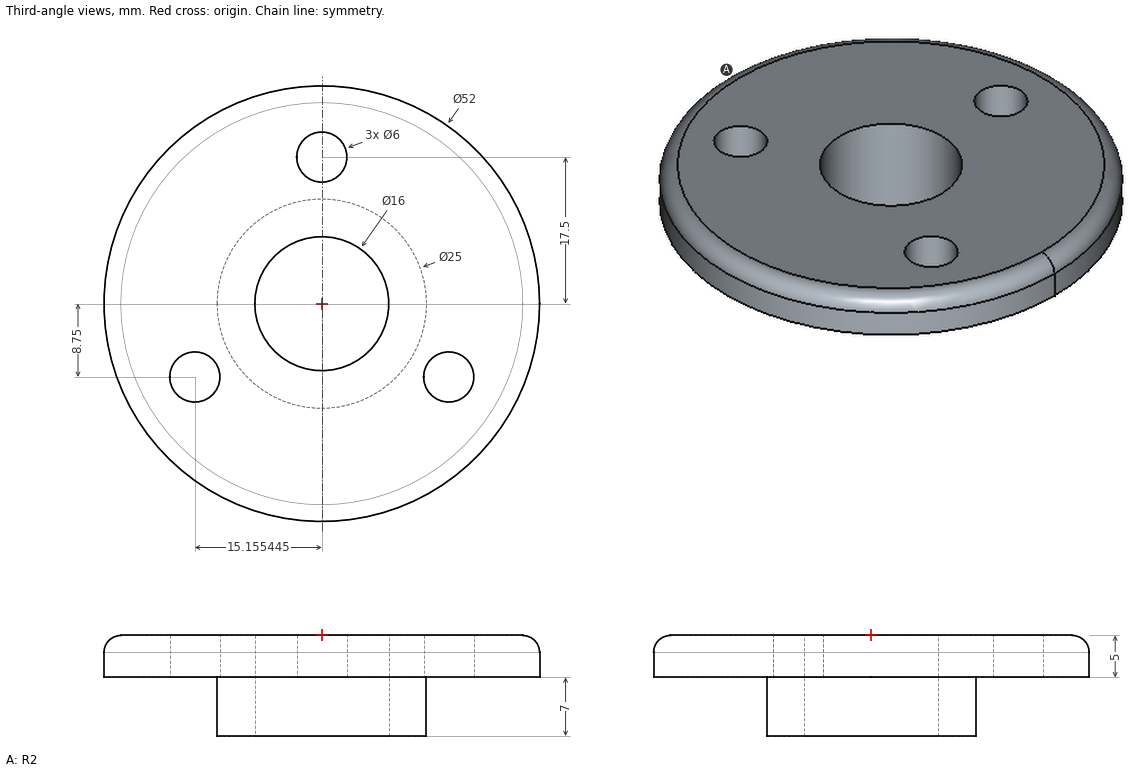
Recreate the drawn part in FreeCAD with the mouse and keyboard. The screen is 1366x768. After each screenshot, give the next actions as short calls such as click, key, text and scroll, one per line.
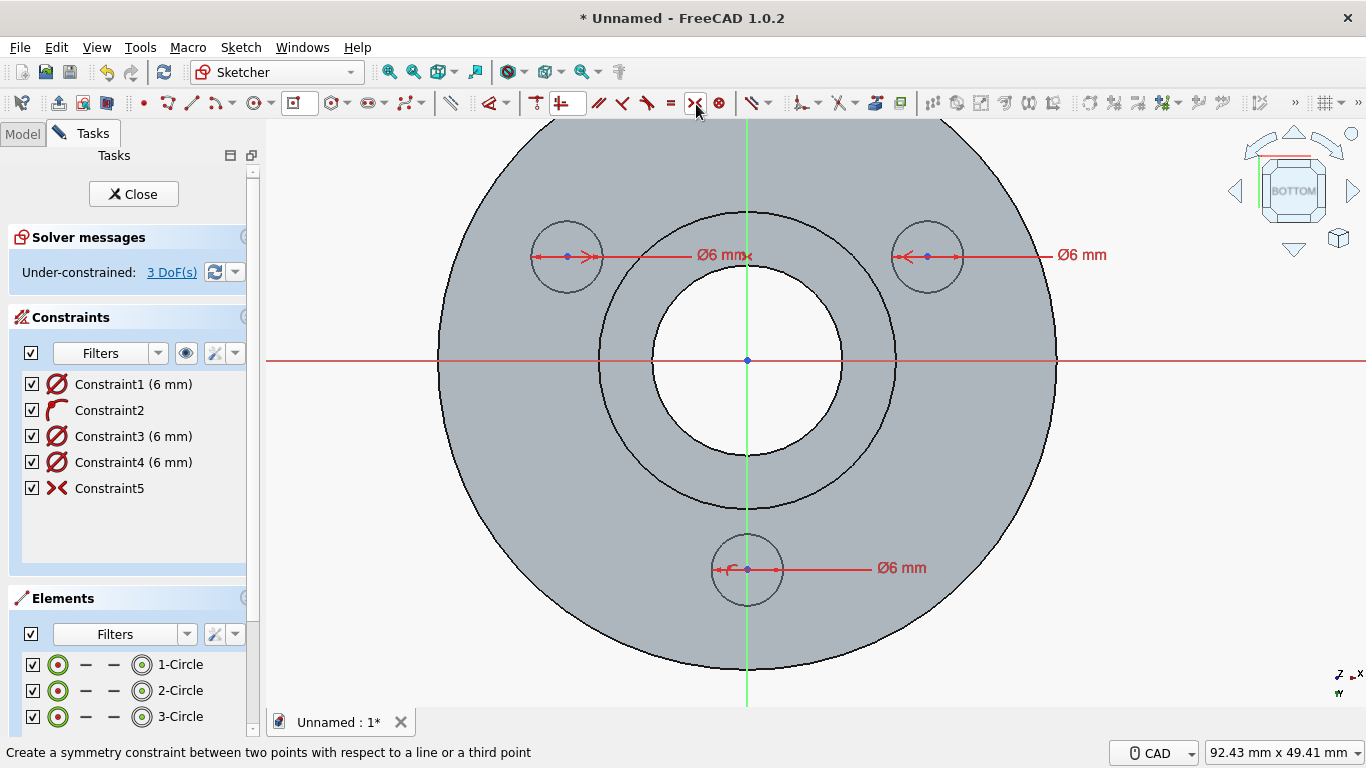
click(490, 104)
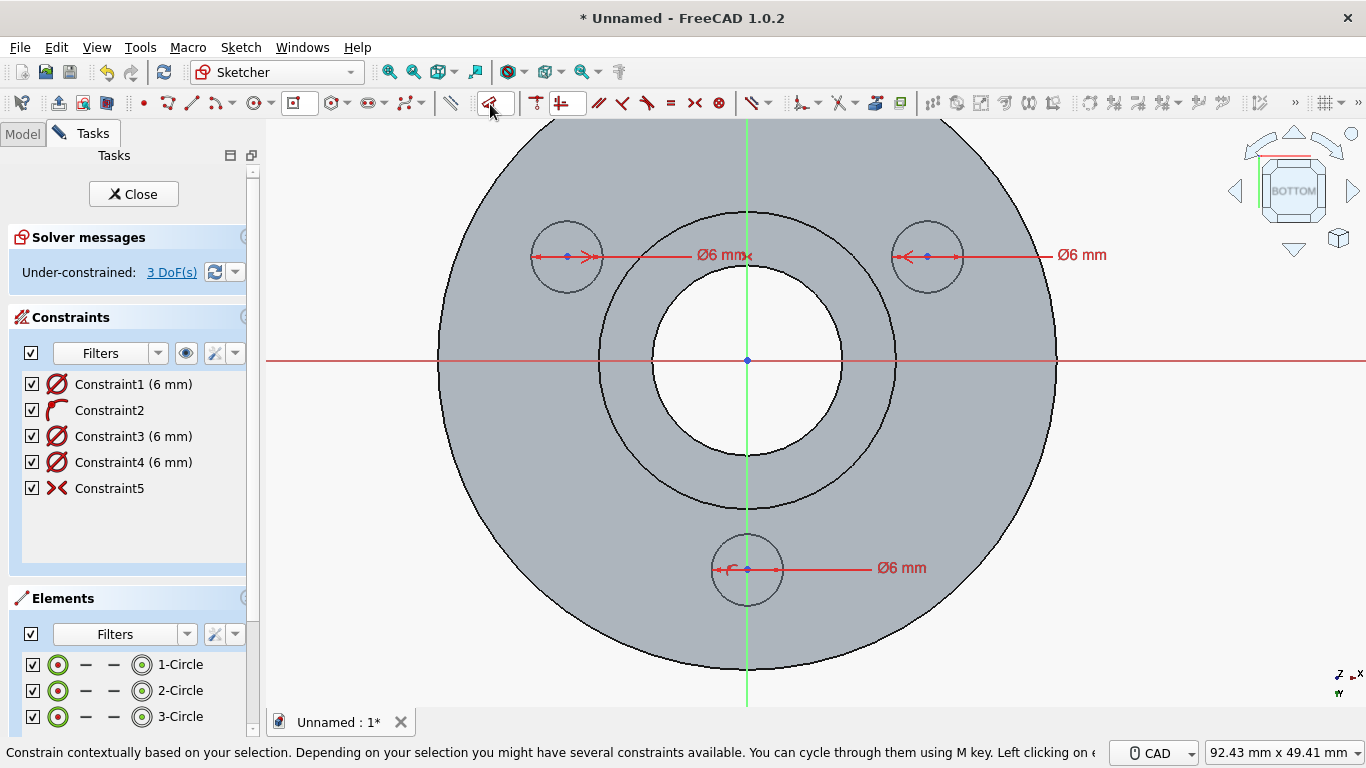
click(747, 570)
click(781, 465)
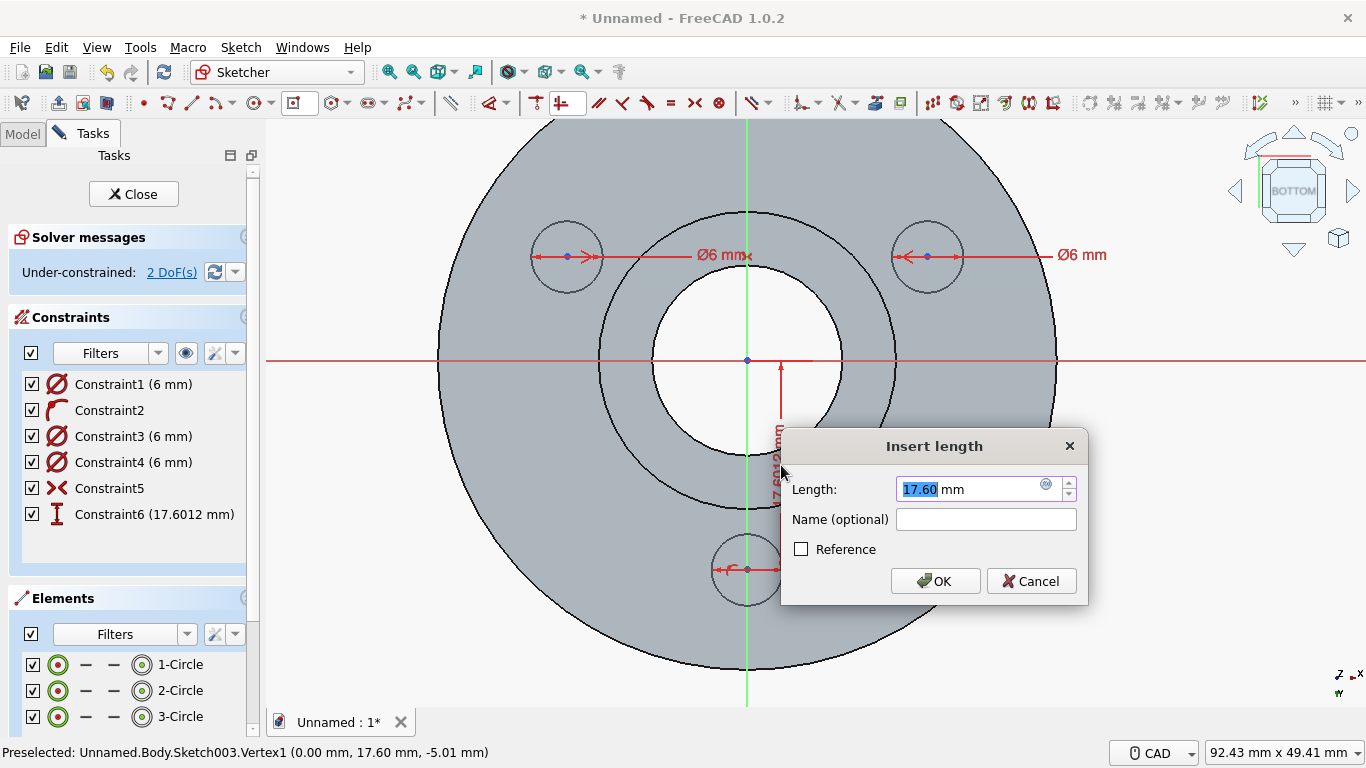
text(17.5)
key(Return)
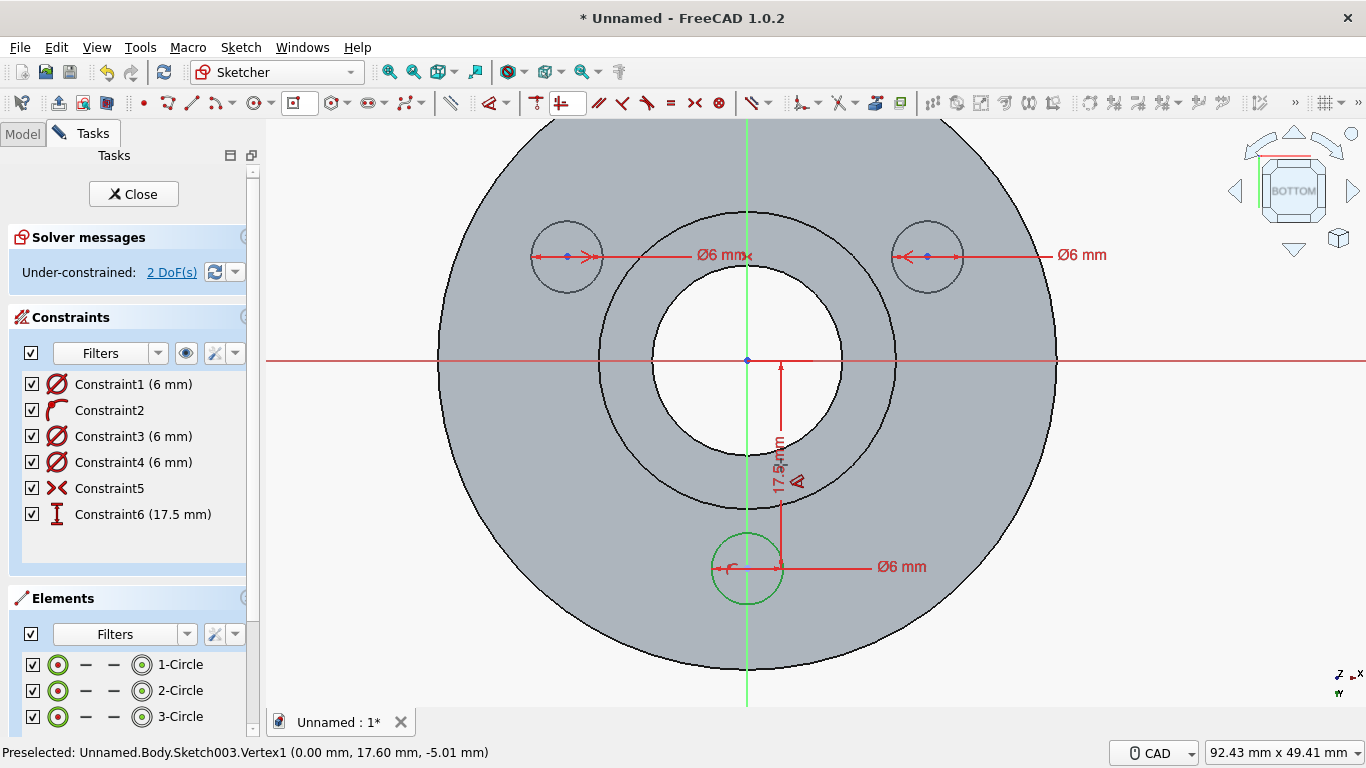
click(567, 257)
click(533, 309)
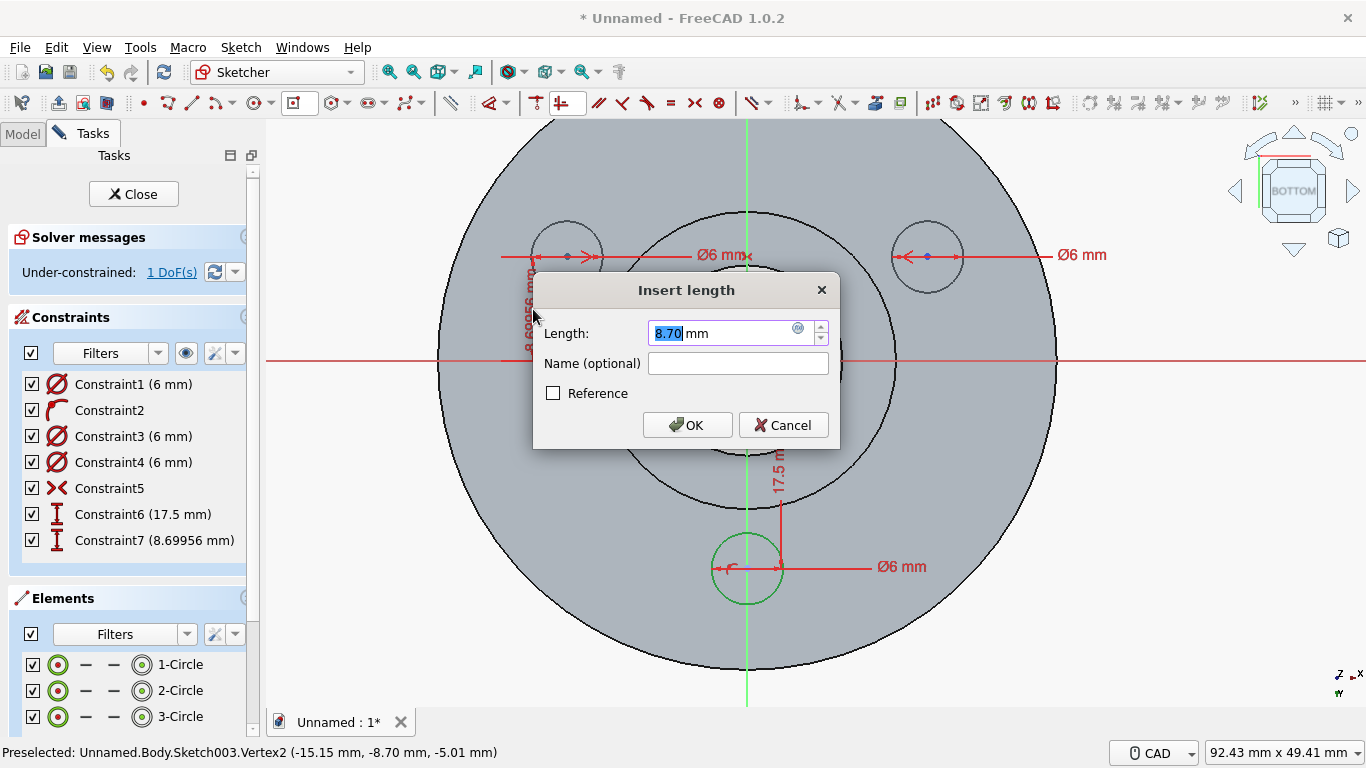
text(8.75)
key(Return)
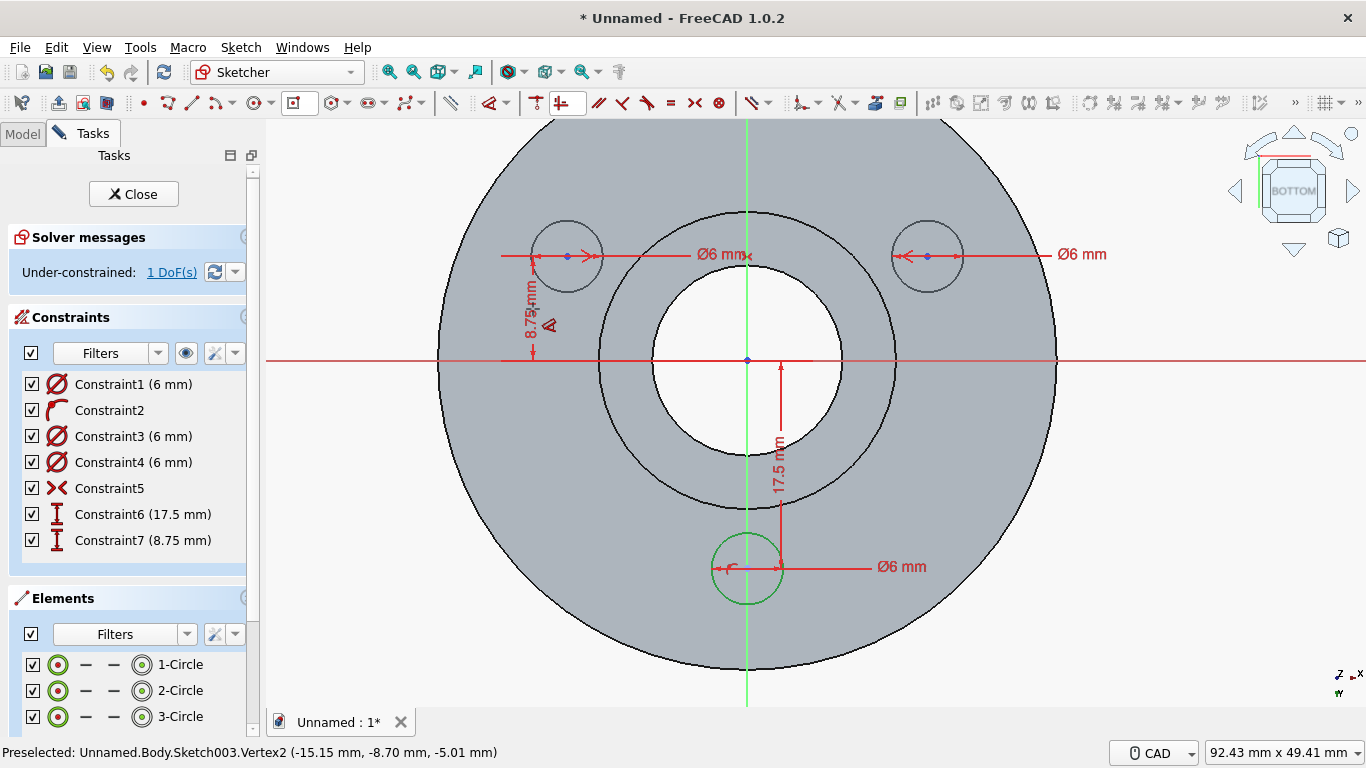
click(567, 256)
click(657, 222)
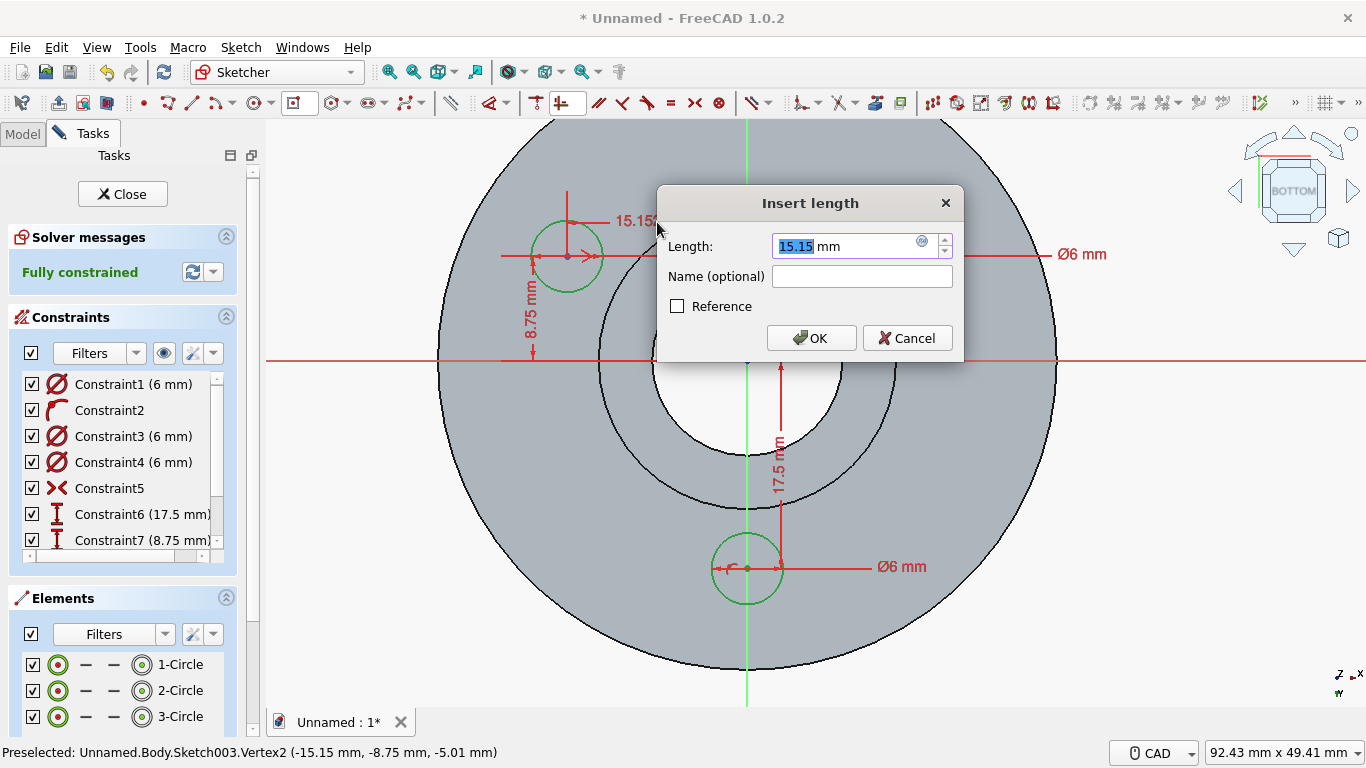
text(15.155445)
key(Return)
key(Escape)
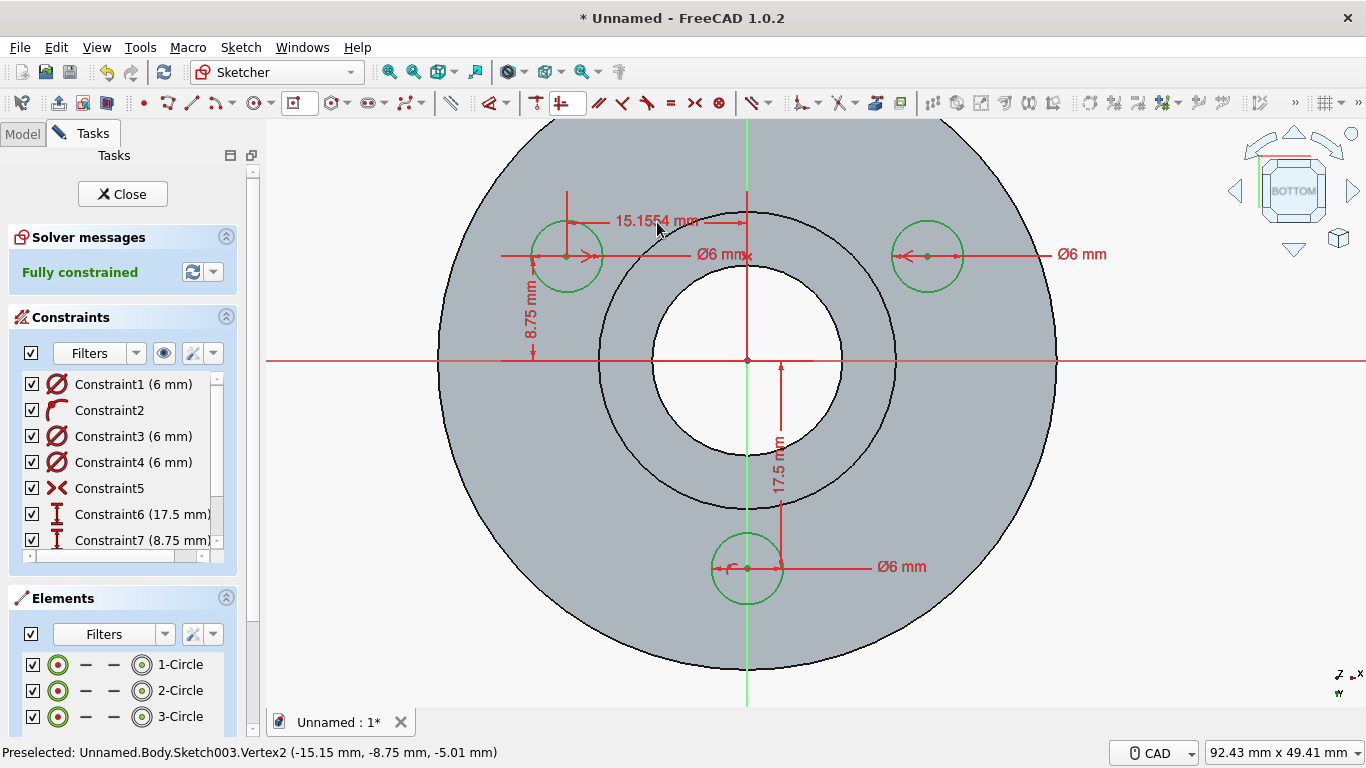
click(123, 194)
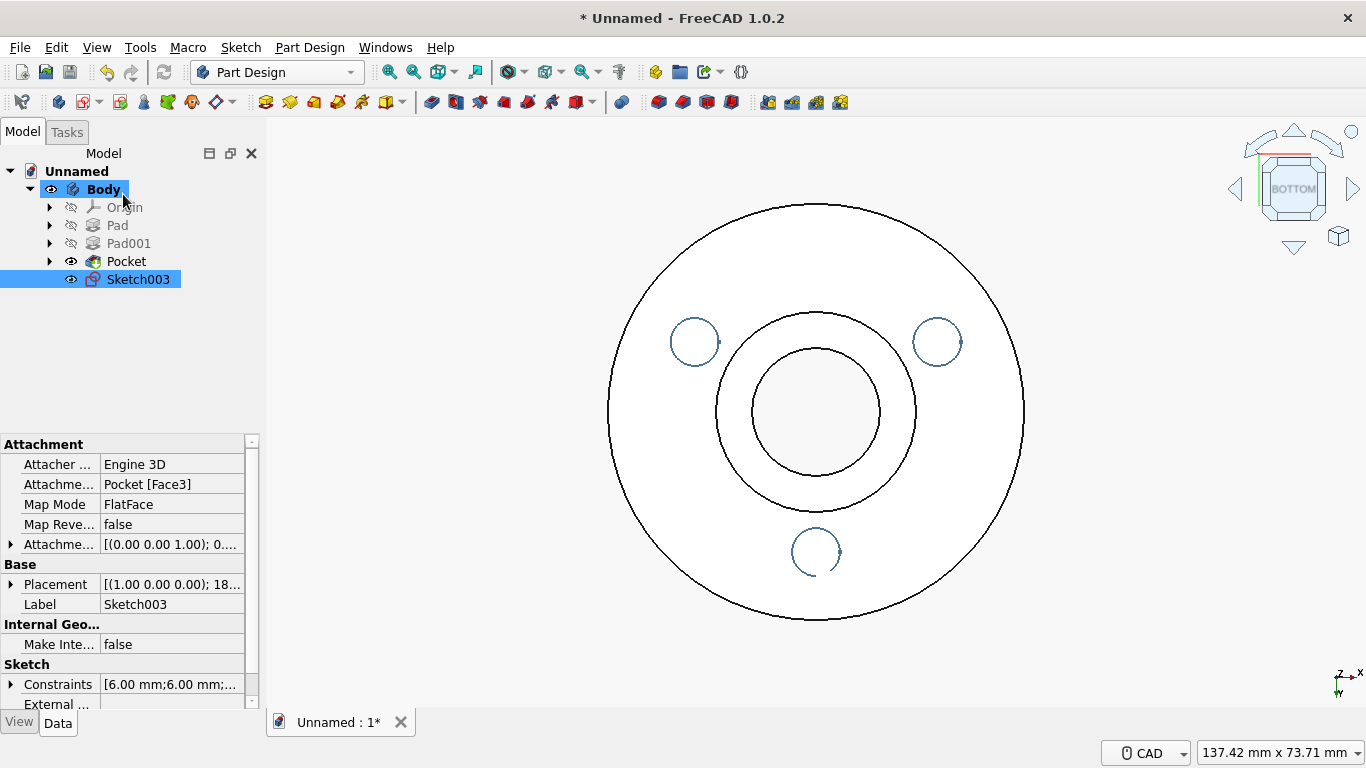
click(432, 102)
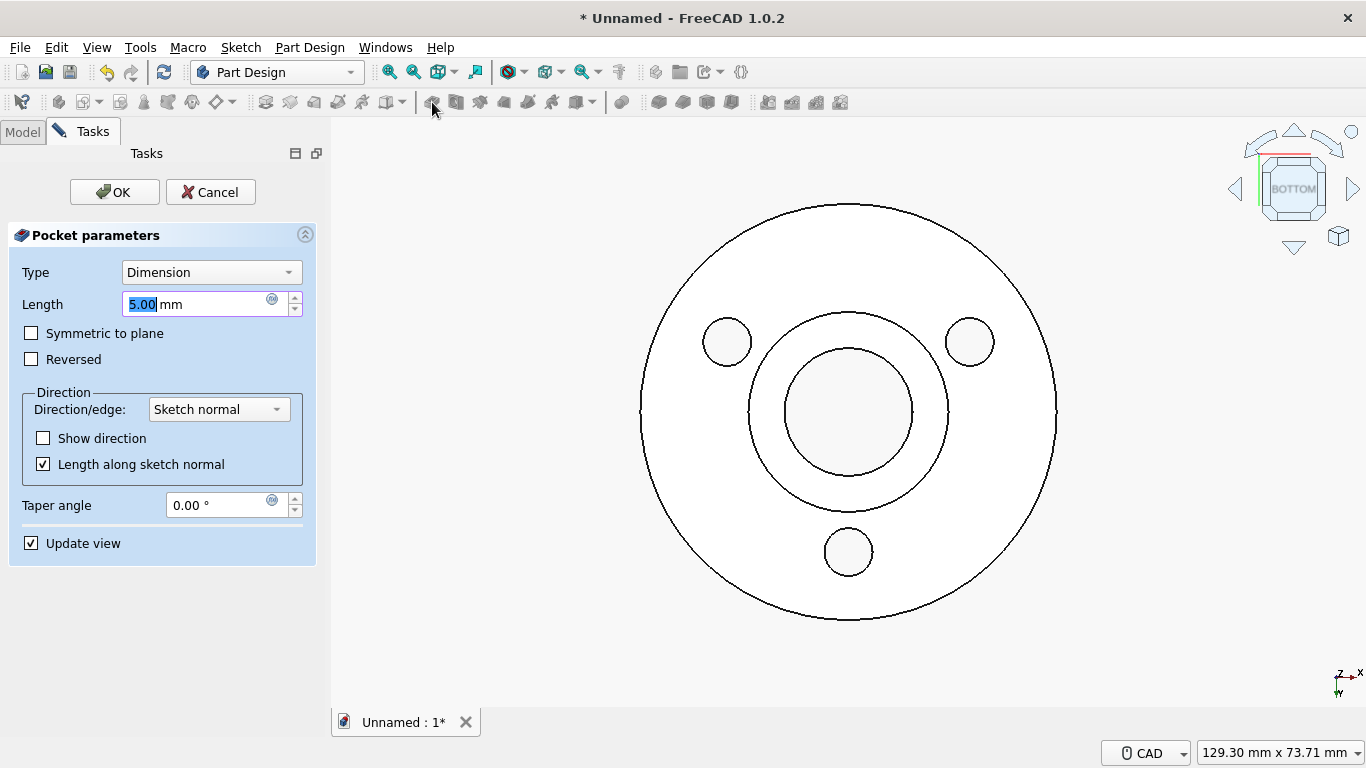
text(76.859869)
key(Tab)